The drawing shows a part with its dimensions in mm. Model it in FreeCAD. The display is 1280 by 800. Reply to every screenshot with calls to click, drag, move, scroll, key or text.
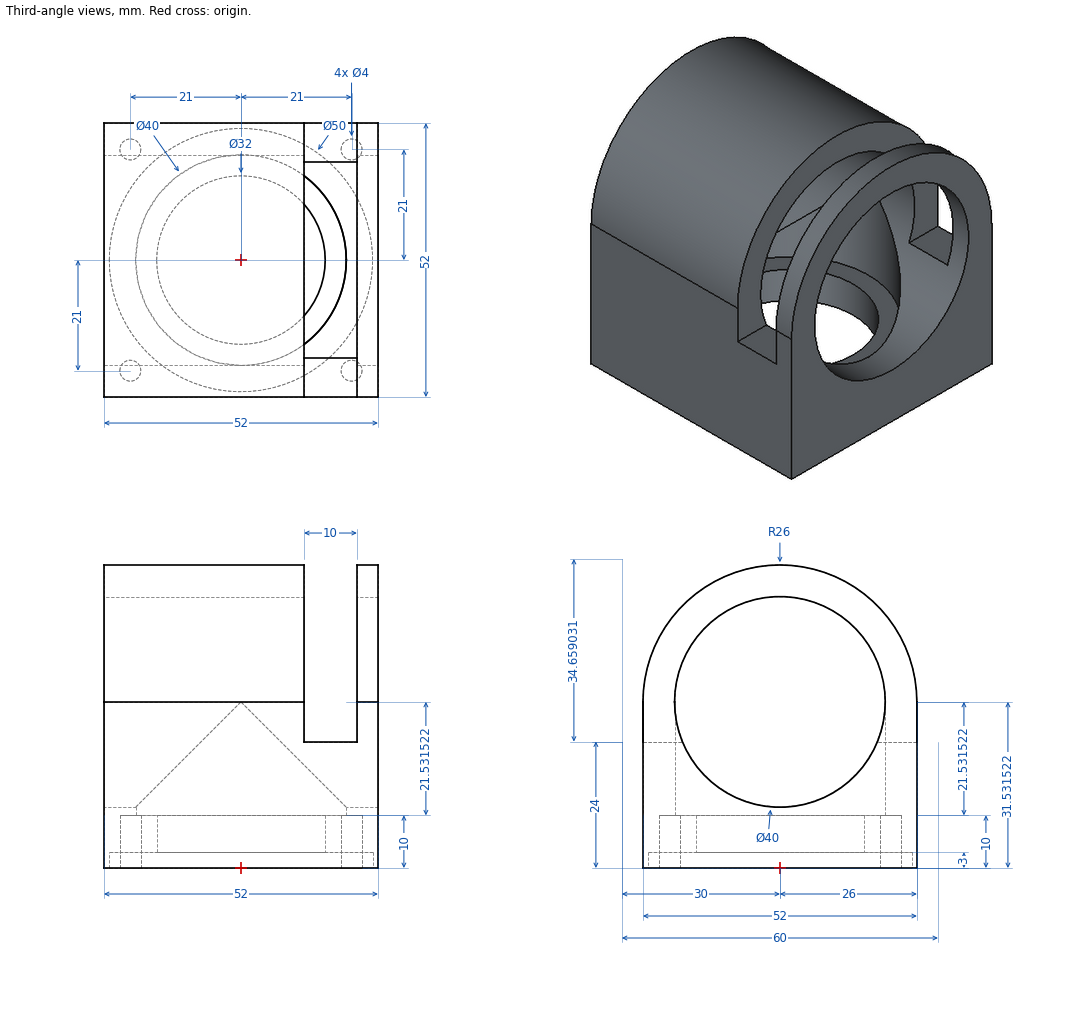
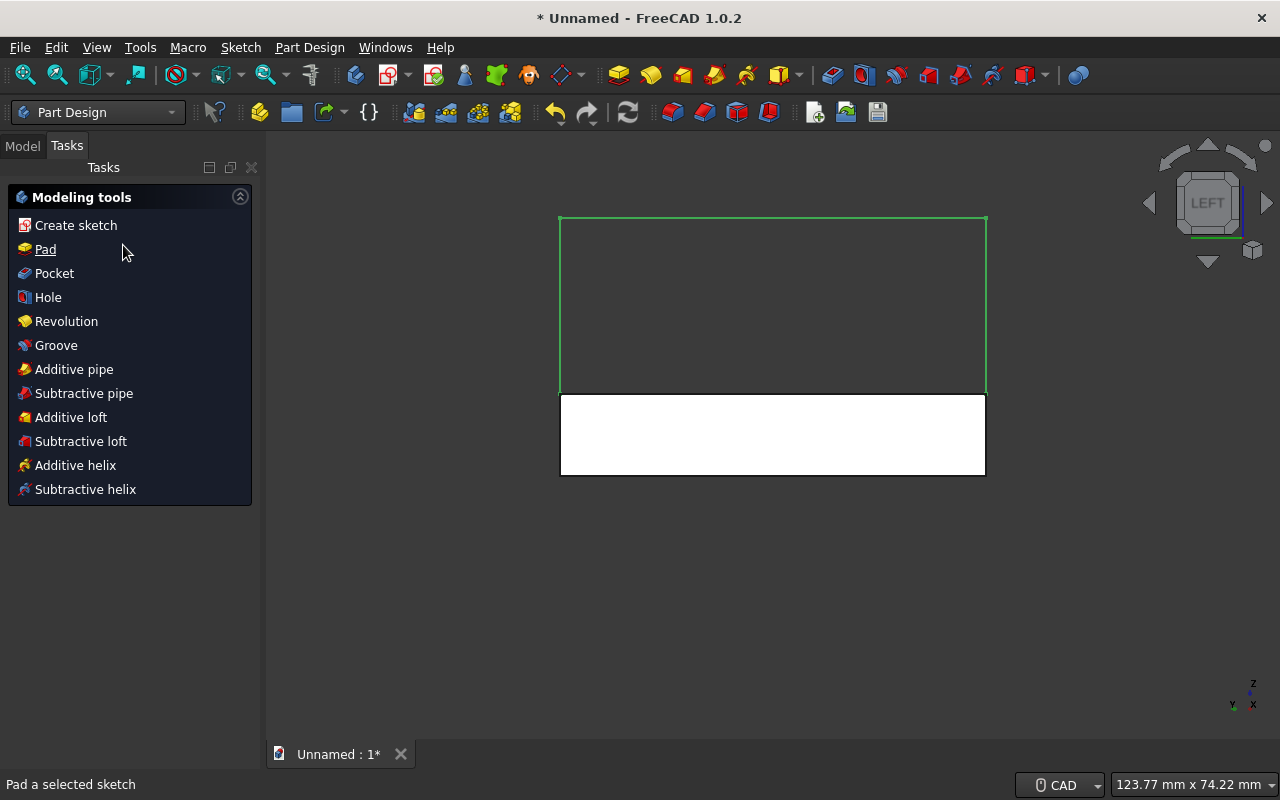
click(620, 76)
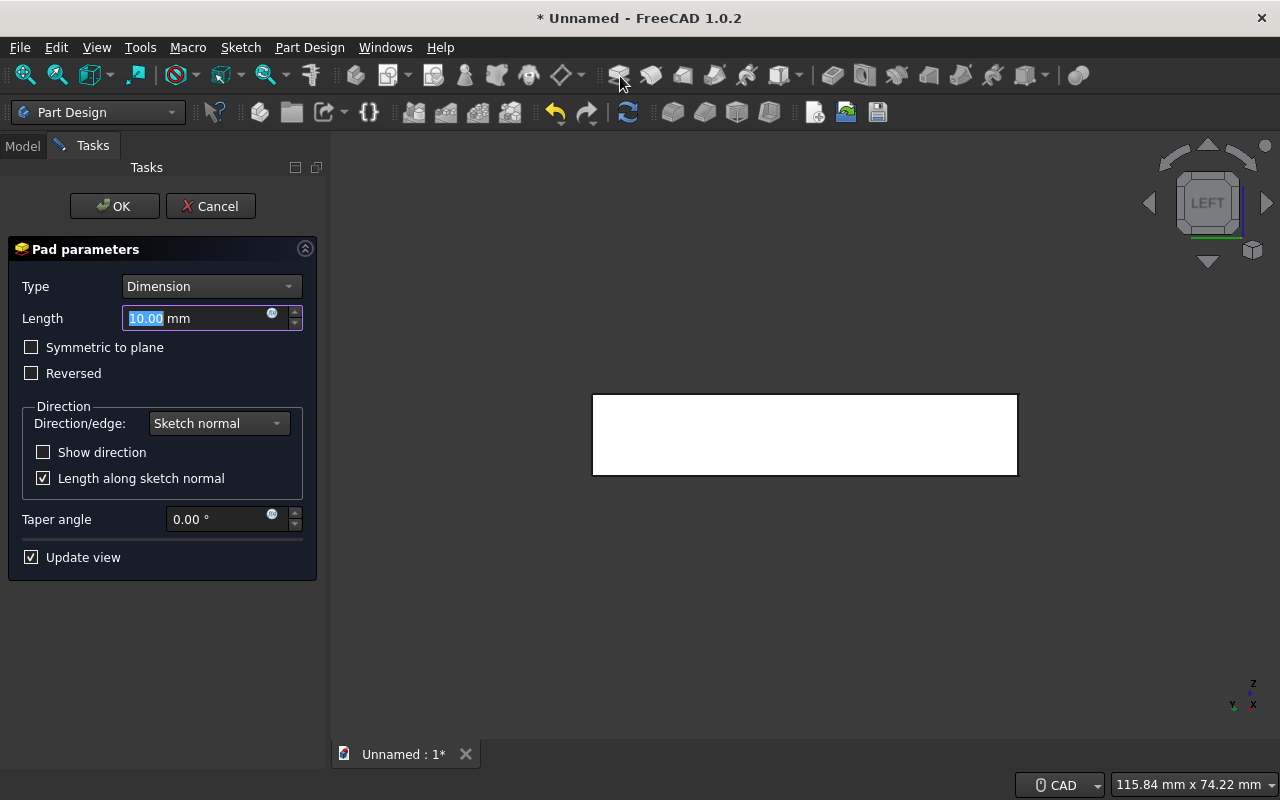
text(52)
key(Tab)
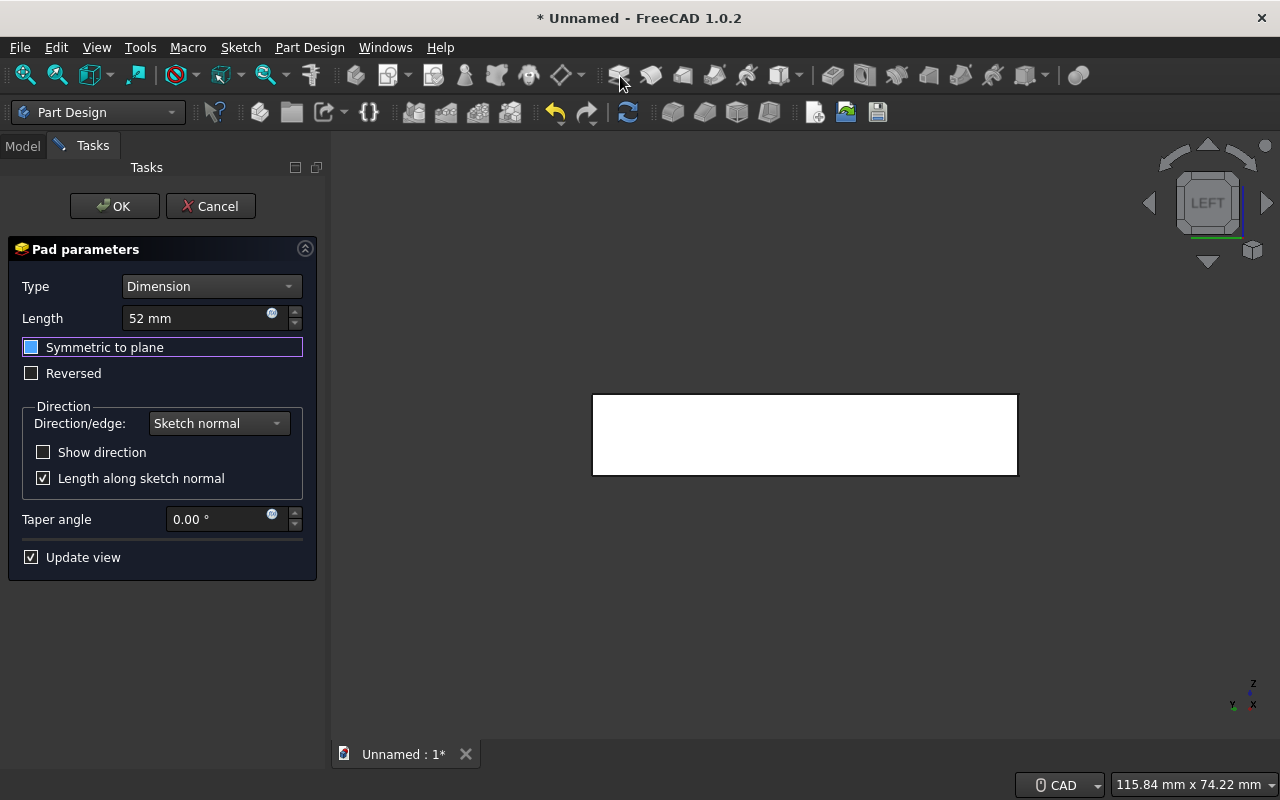
click(30, 373)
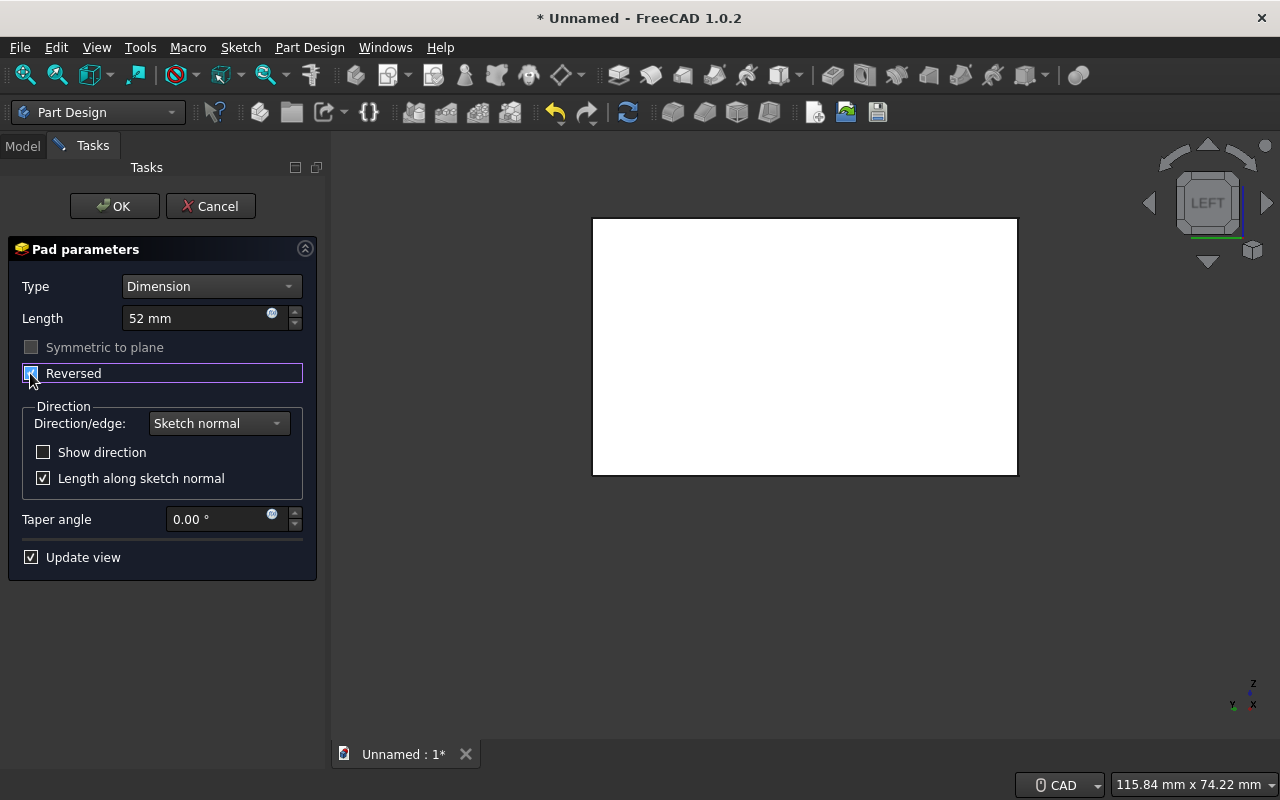
click(115, 206)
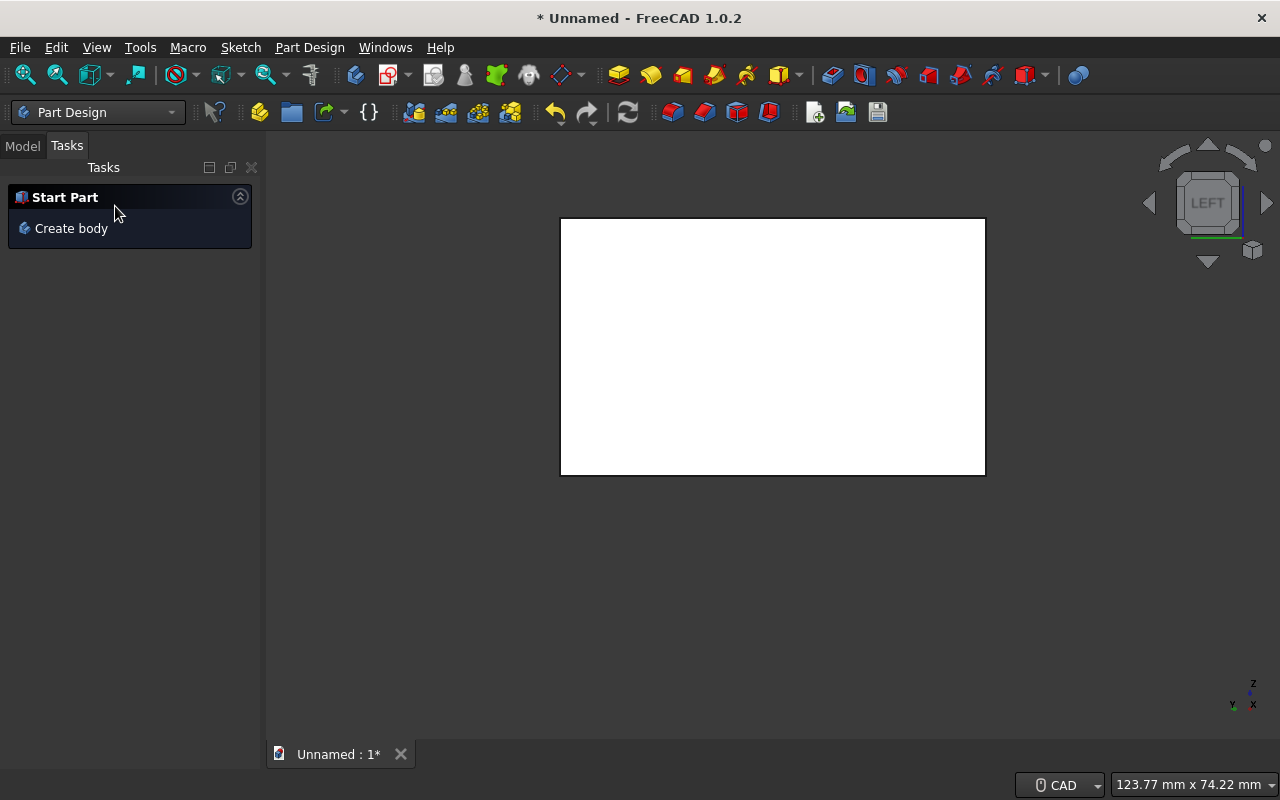
click(26, 76)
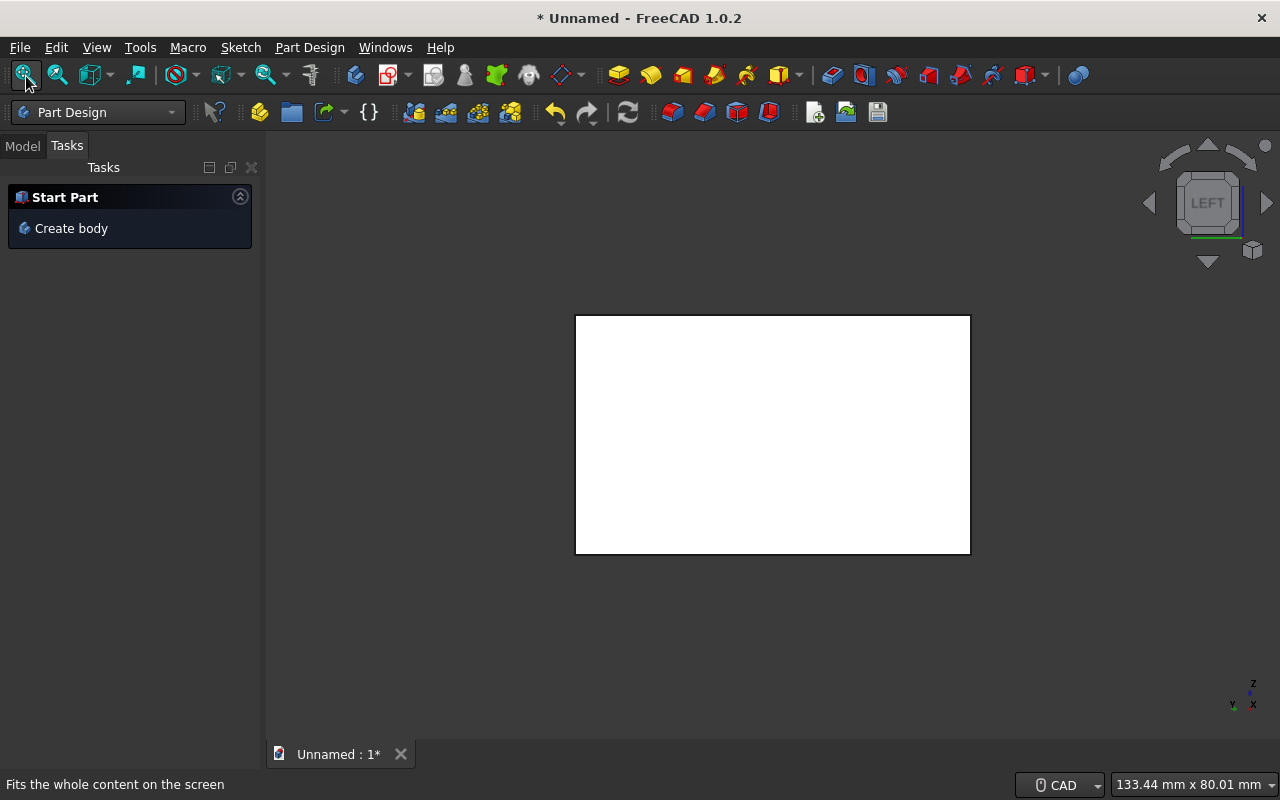
key(0)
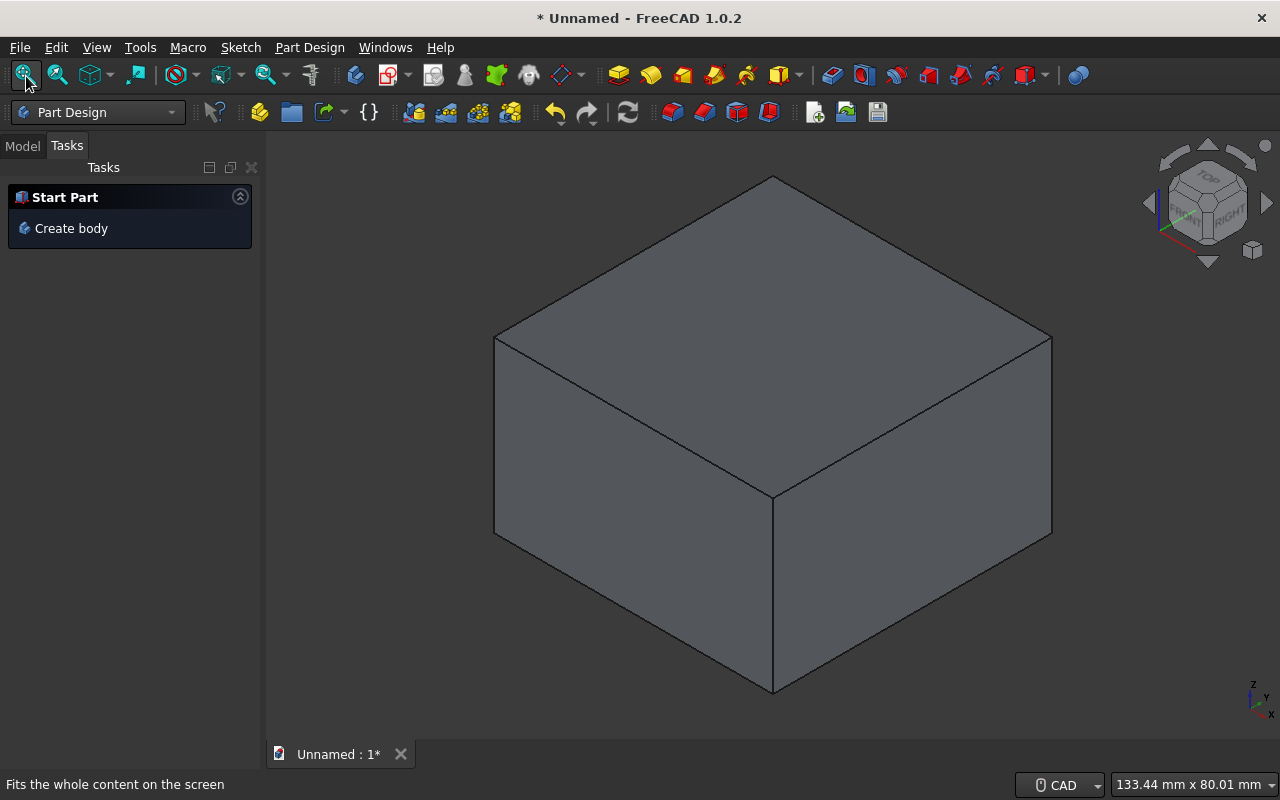
click(773, 336)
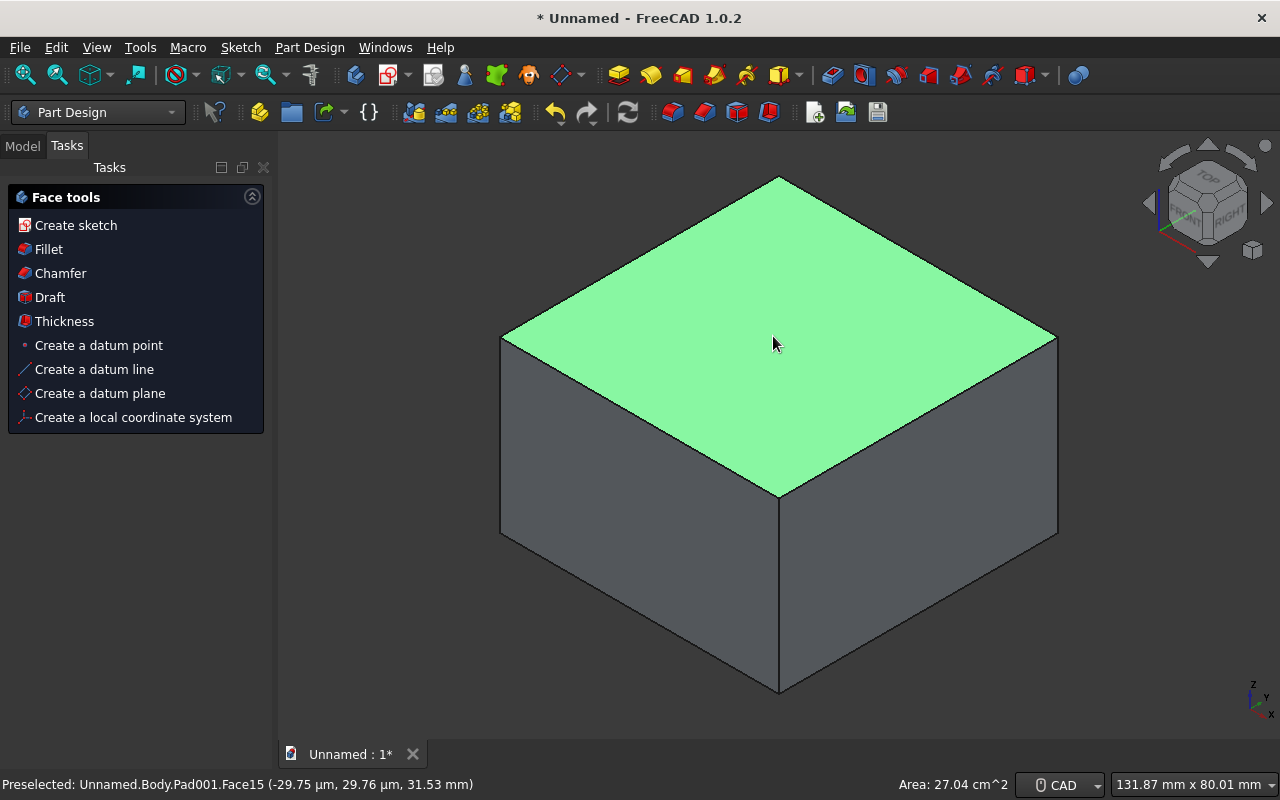
click(388, 76)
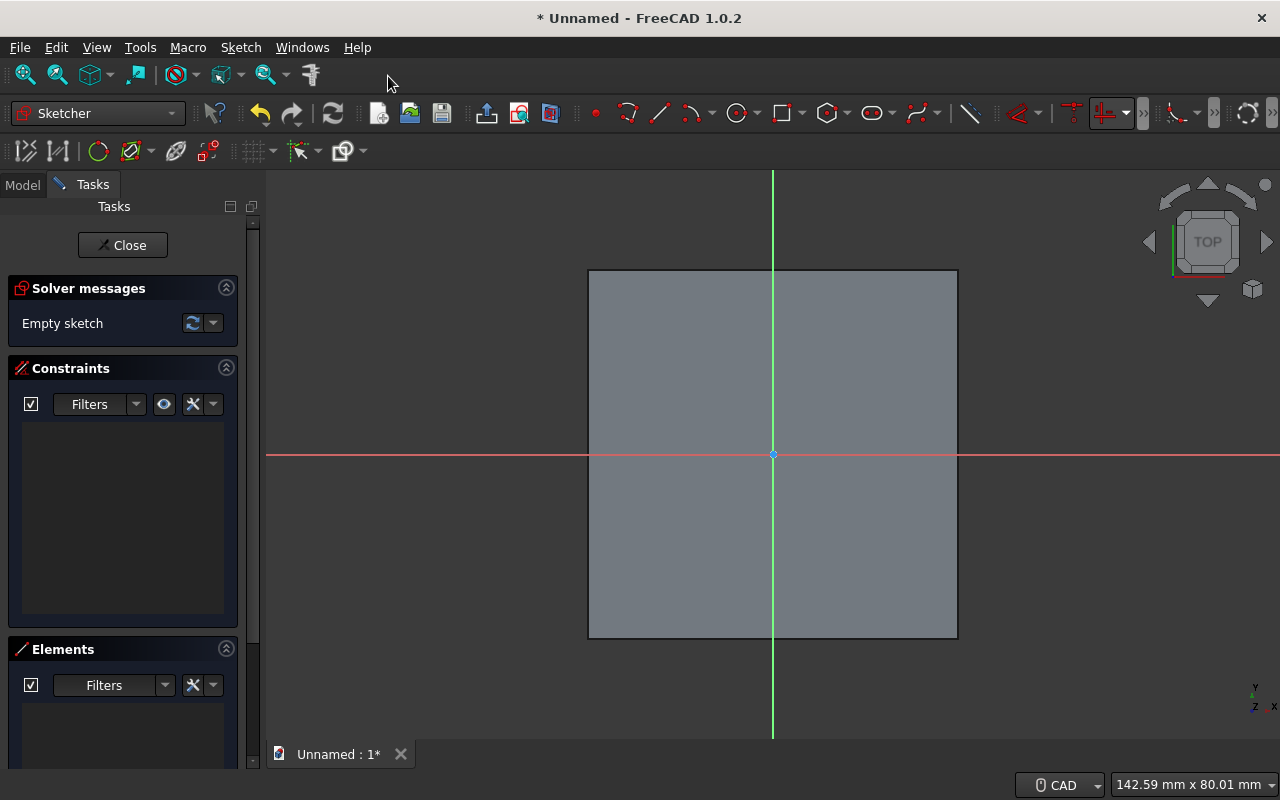
click(738, 114)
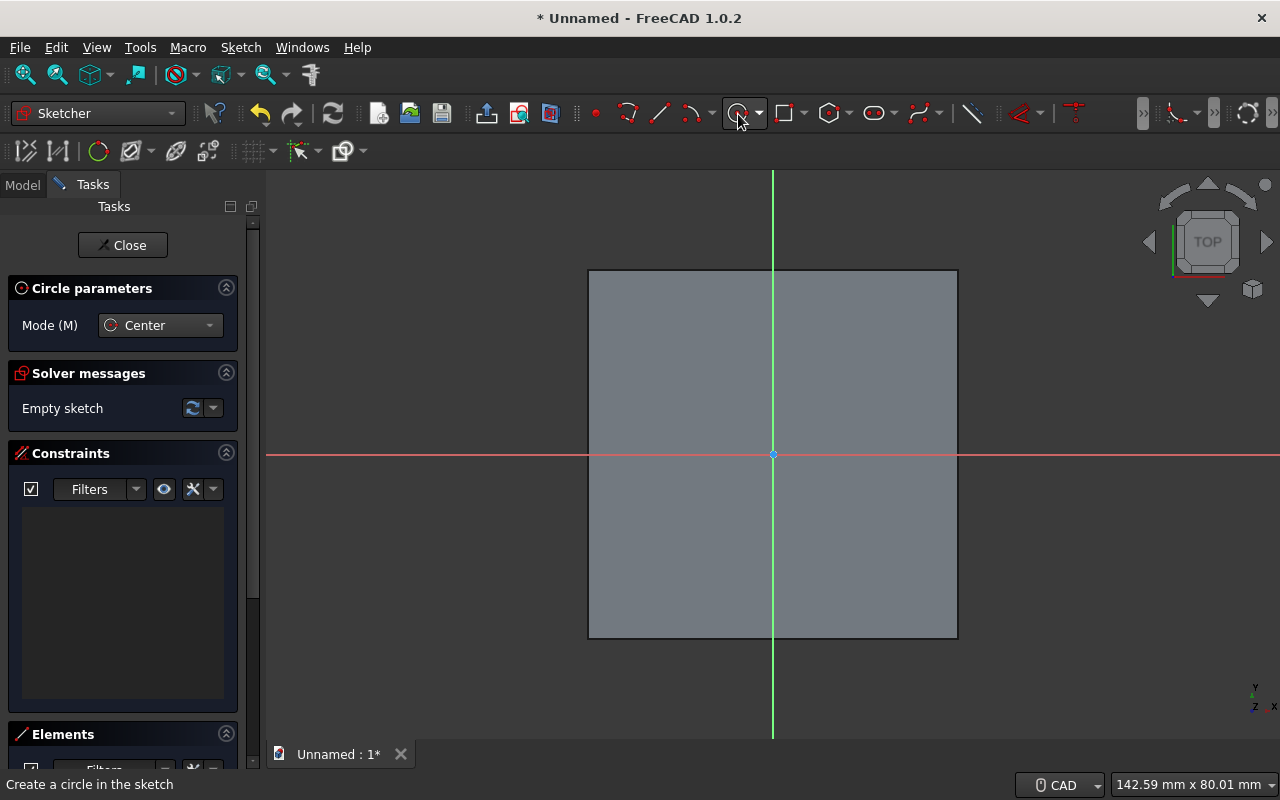
click(773, 455)
click(874, 354)
key(Escape)